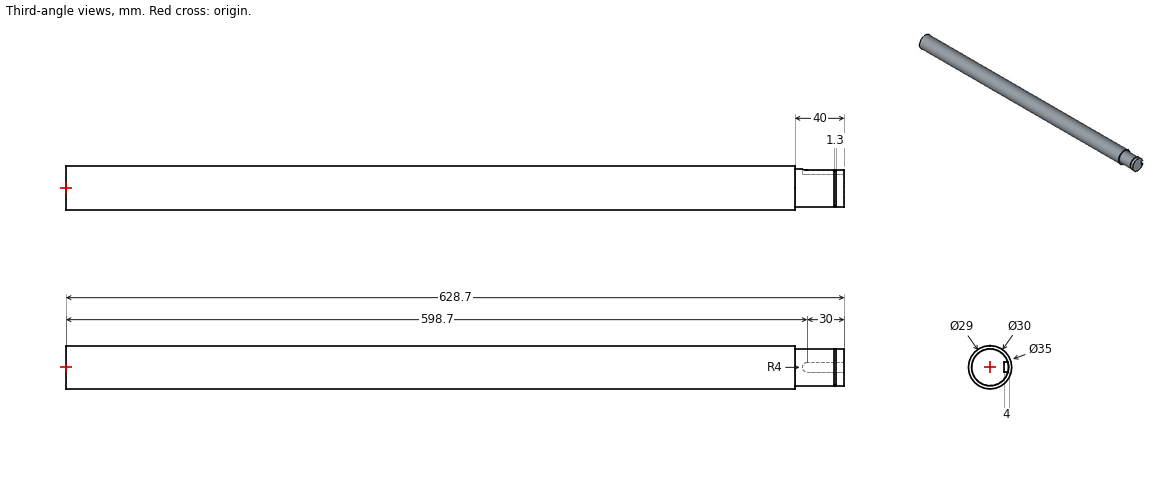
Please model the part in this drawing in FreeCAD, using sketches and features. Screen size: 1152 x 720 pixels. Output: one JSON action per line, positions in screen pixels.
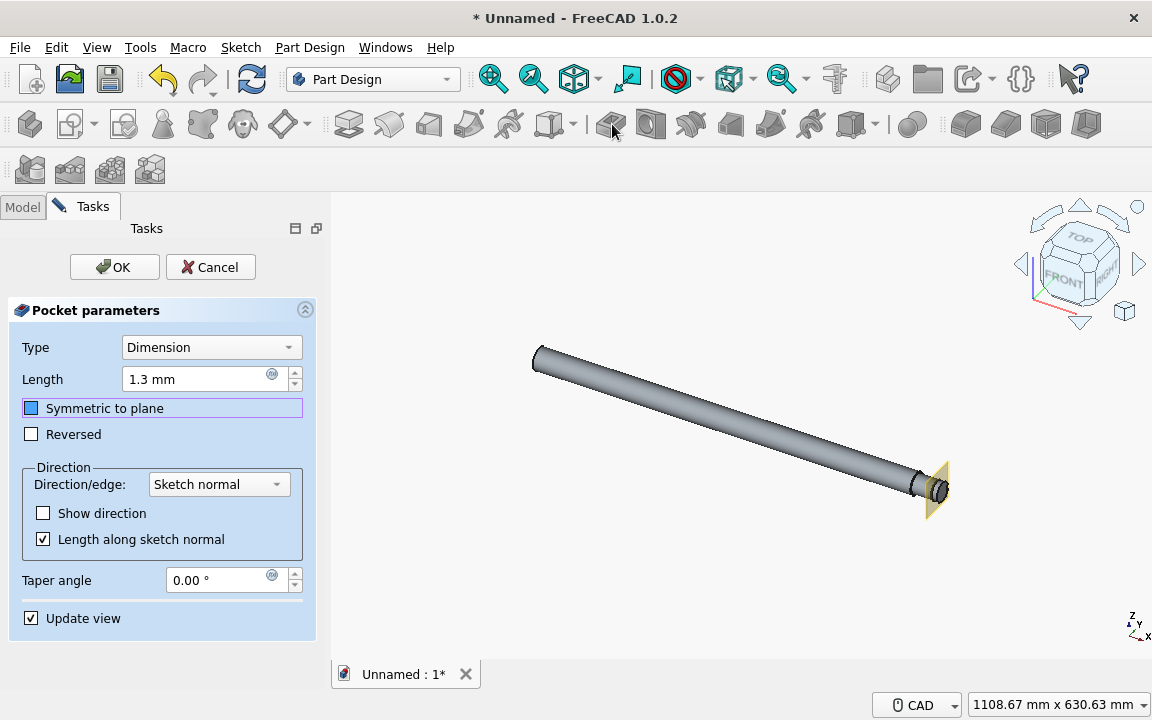
{"action": "left_click", "coordinate": [30, 434]}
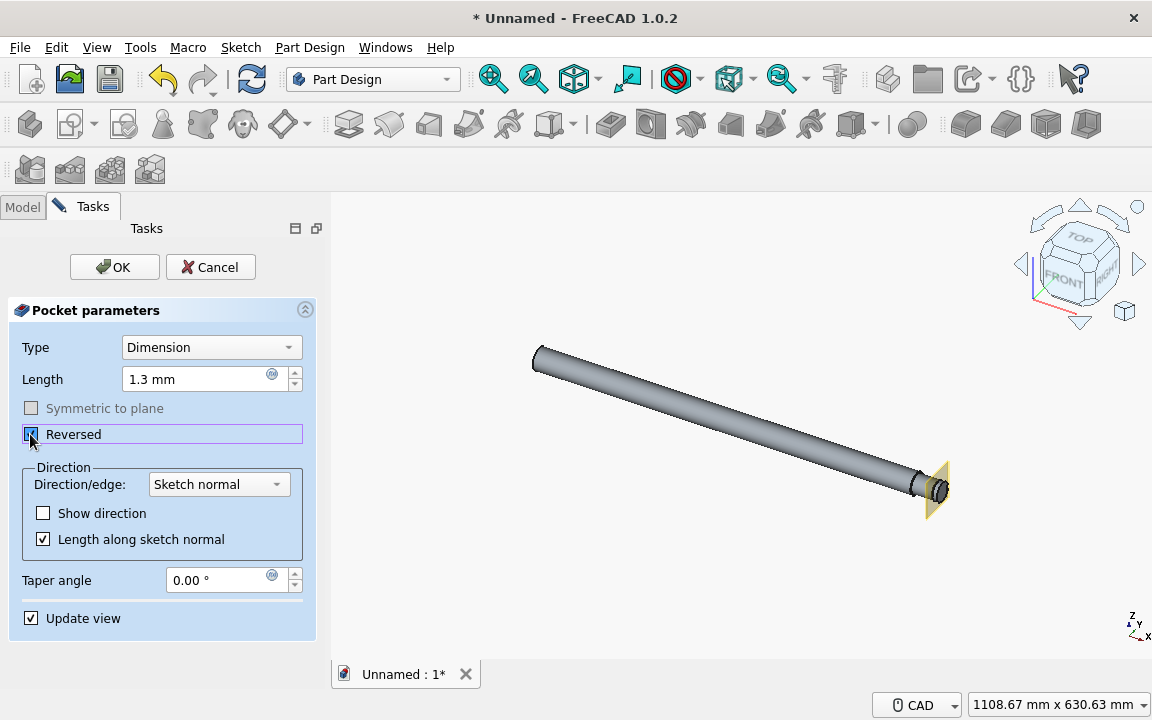
{"action": "left_click", "coordinate": [115, 267]}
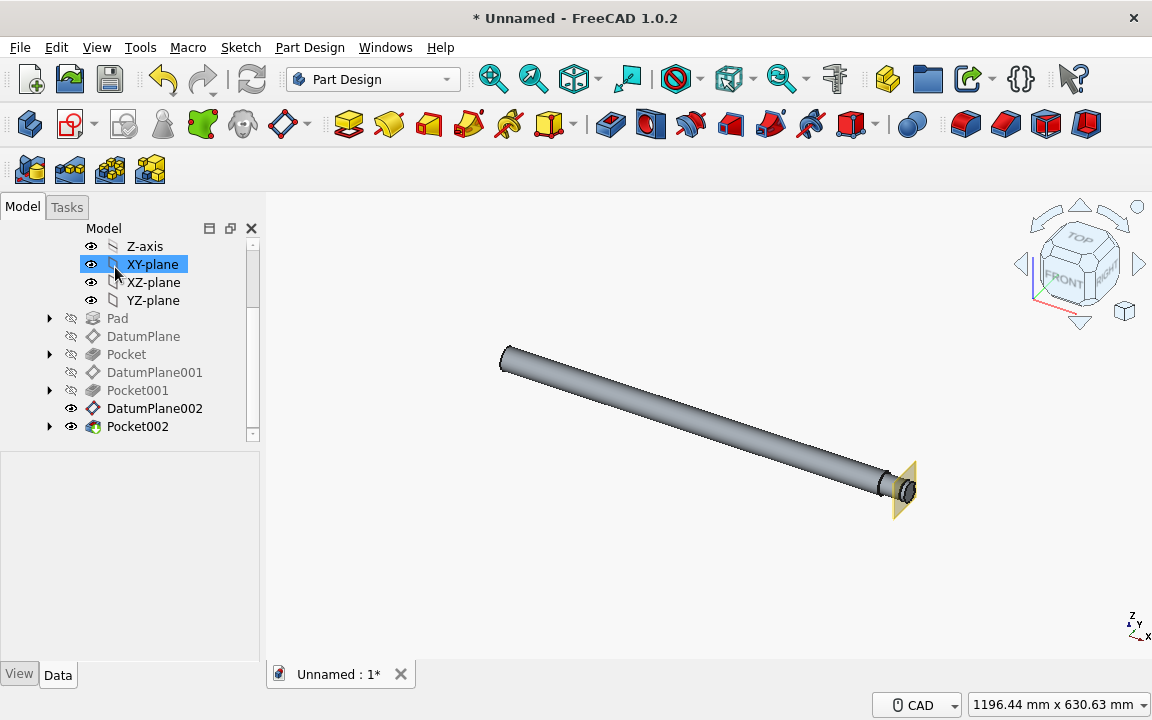
{"action": "left_click", "coordinate": [116, 408]}
{"action": "key", "text": "space"}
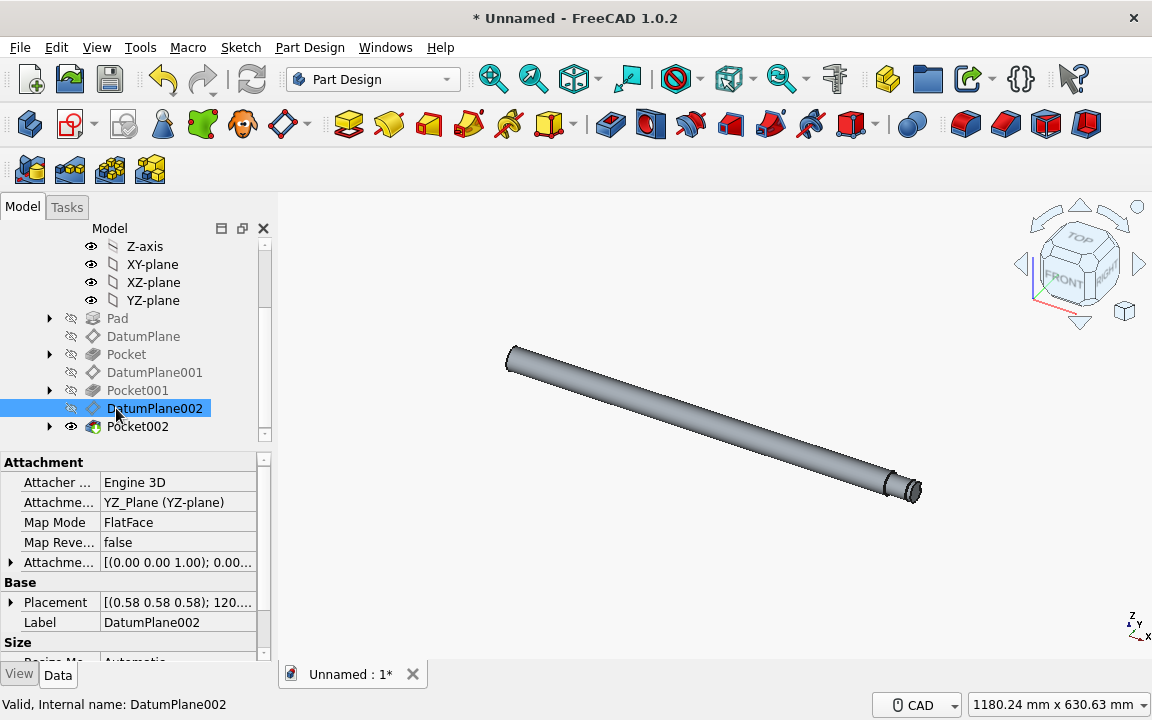
{"action": "key", "text": "0"}